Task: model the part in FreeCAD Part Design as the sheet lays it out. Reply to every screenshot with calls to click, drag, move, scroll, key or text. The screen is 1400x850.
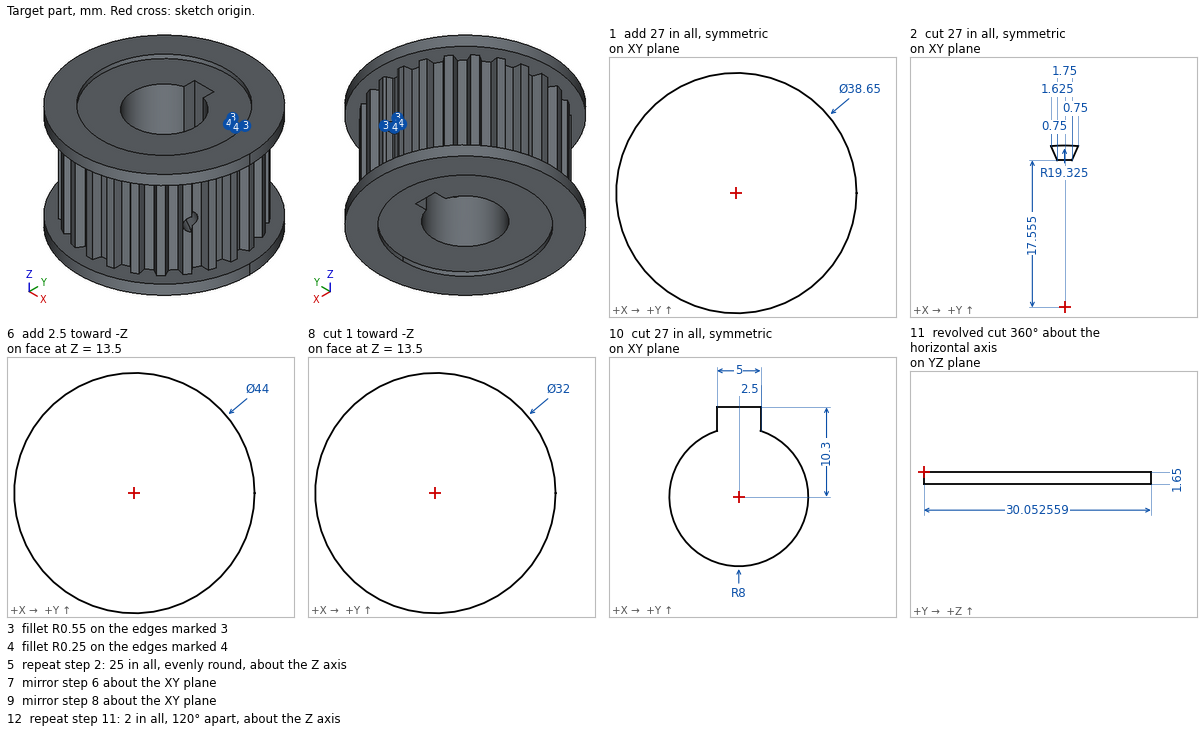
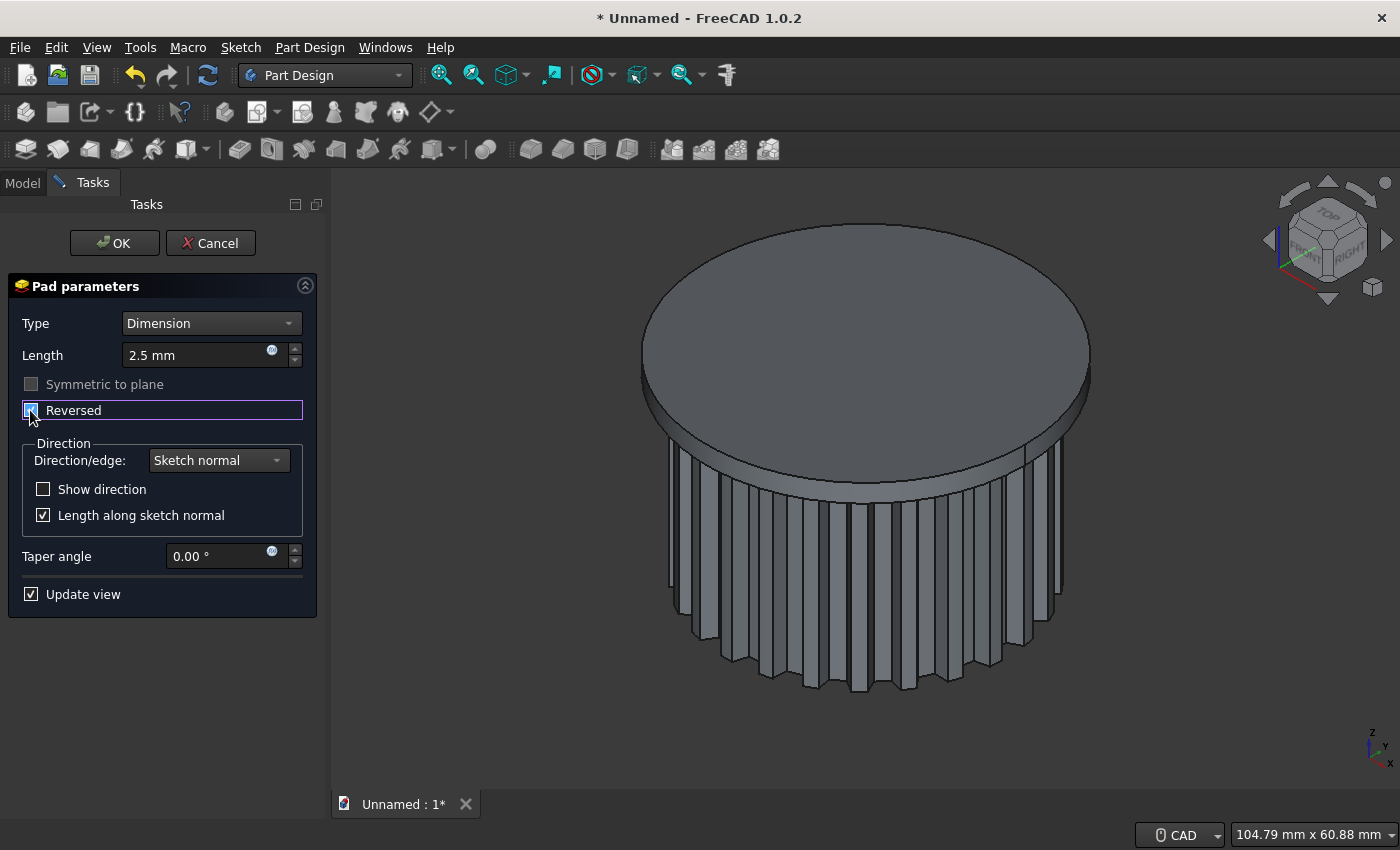
click(115, 243)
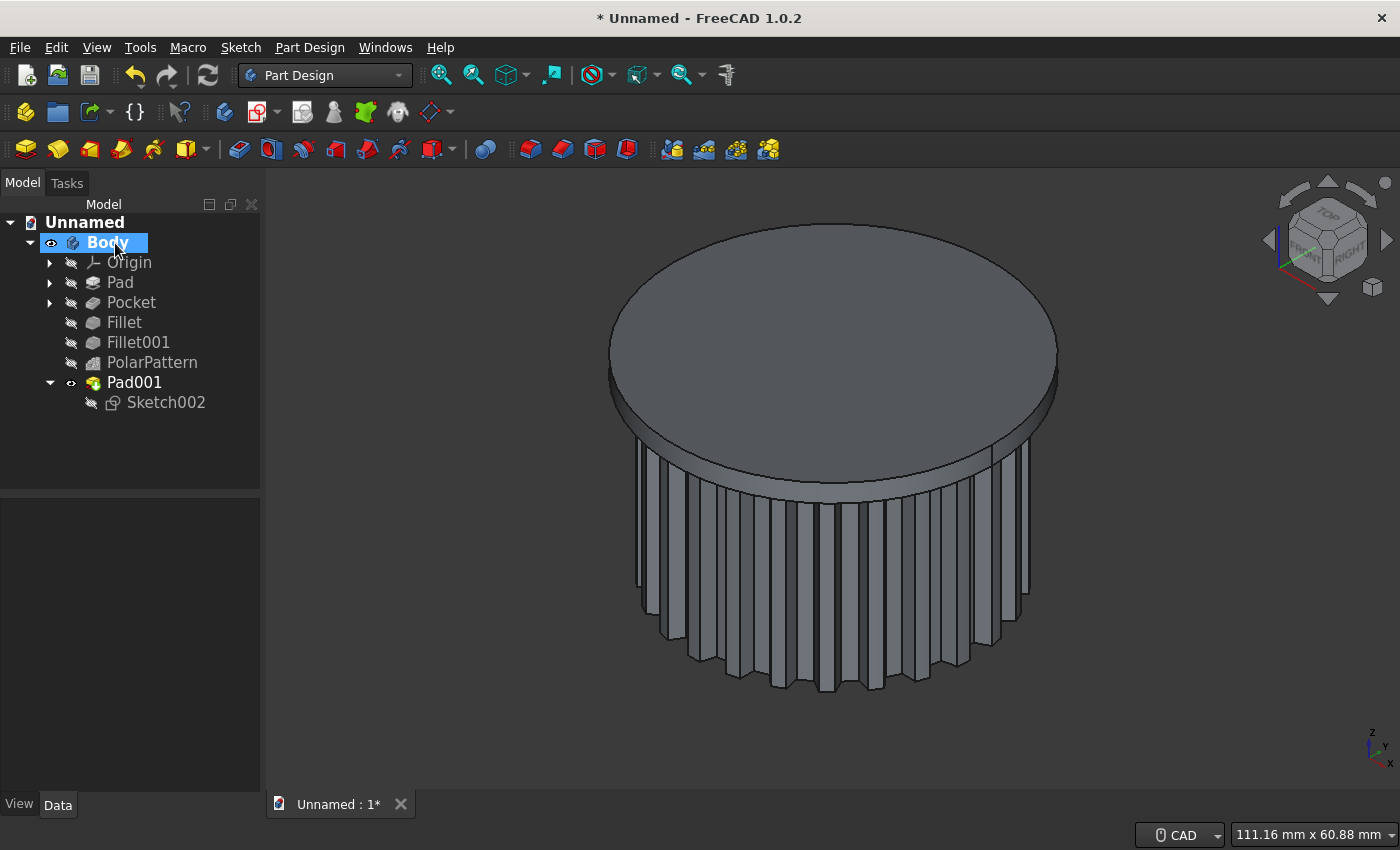
click(116, 383)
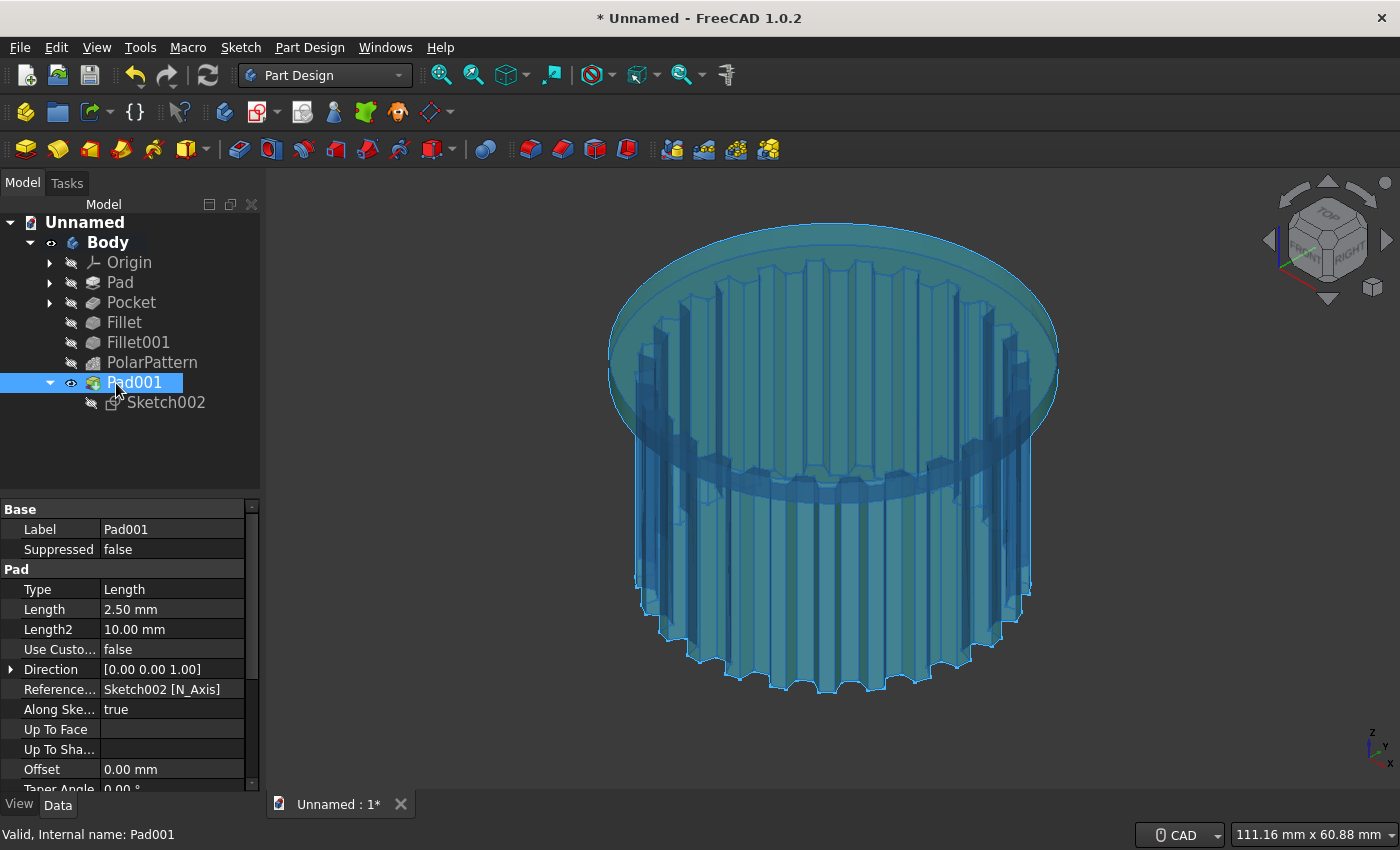
click(672, 150)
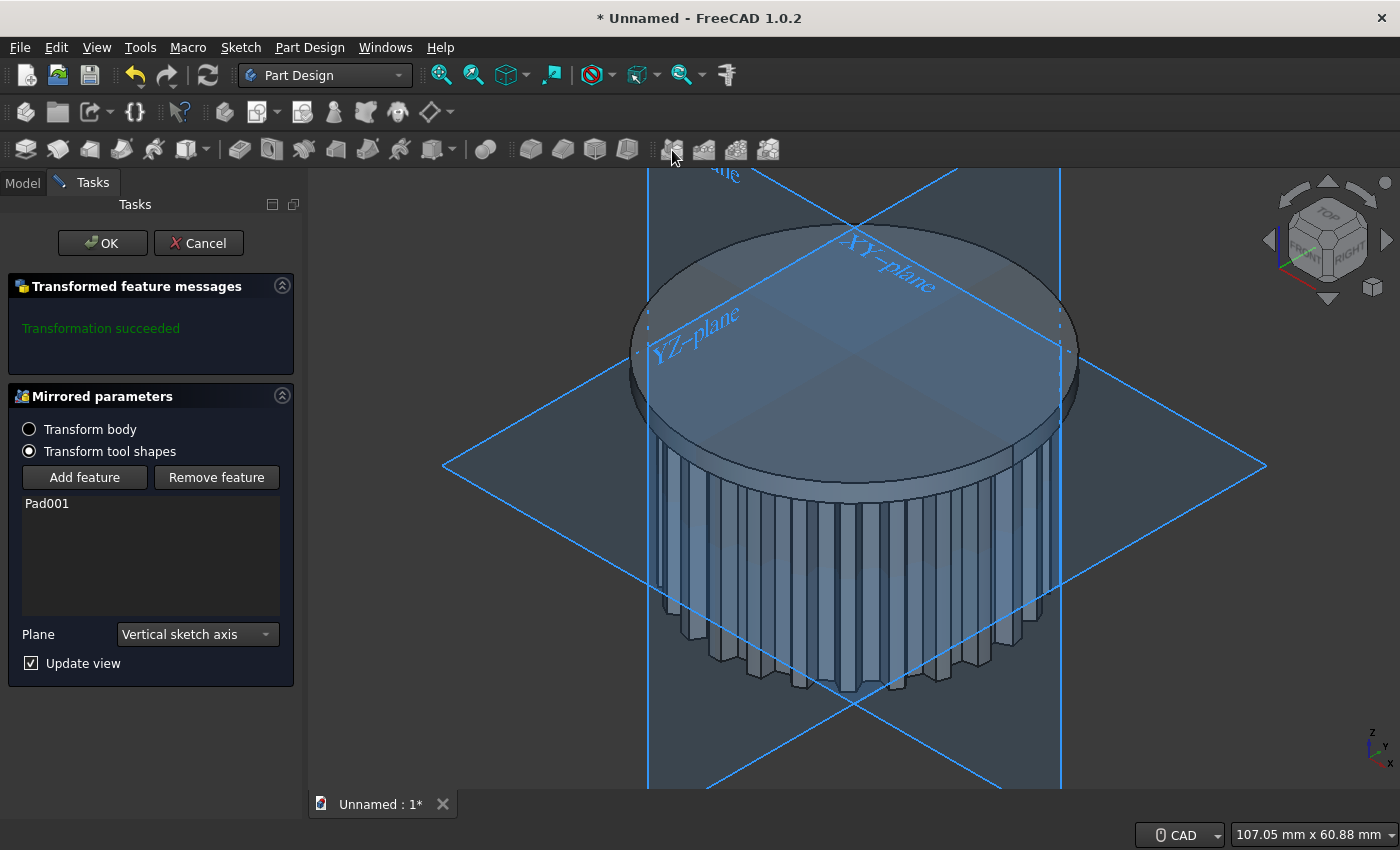
click(198, 634)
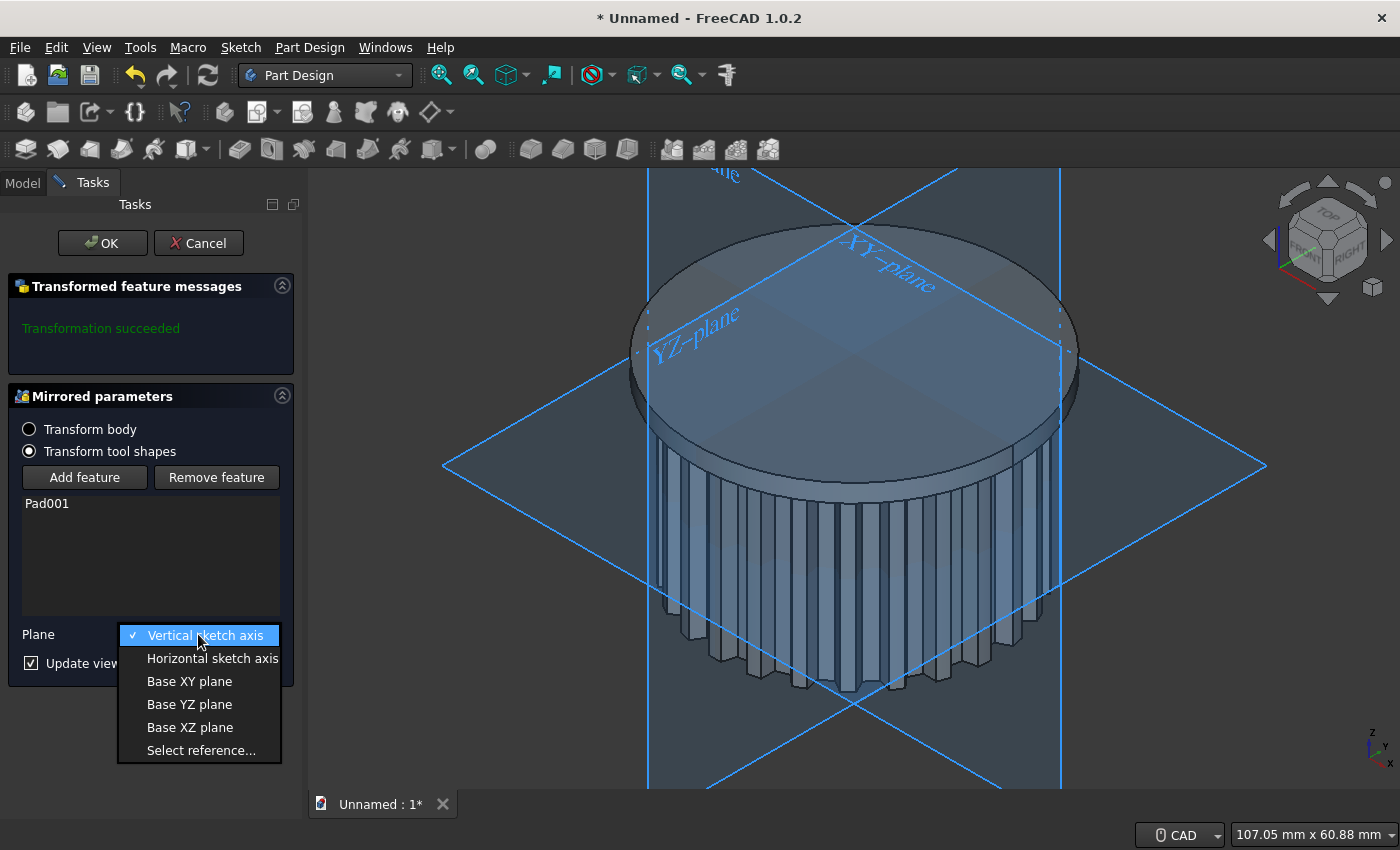
click(198, 682)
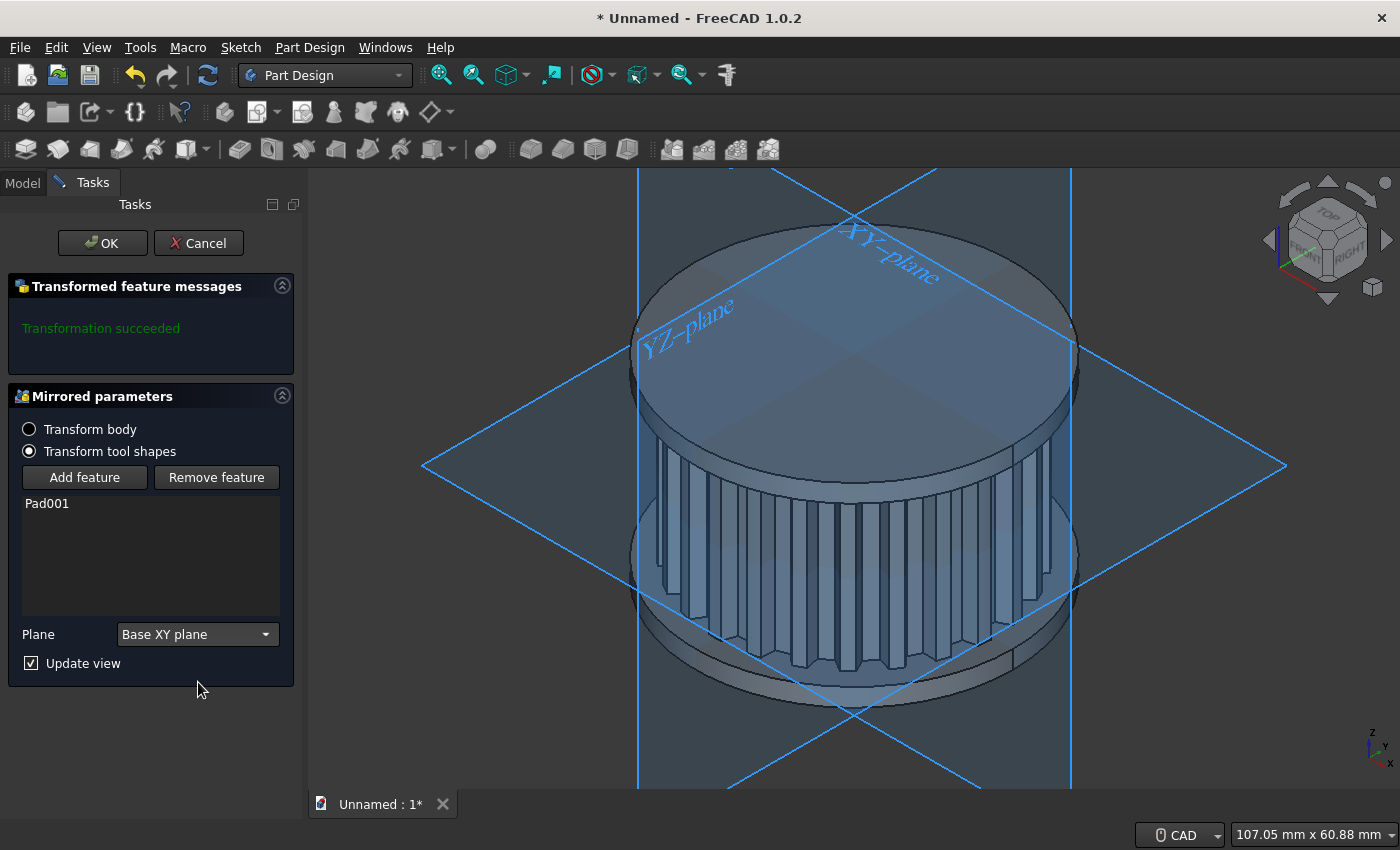
click(103, 243)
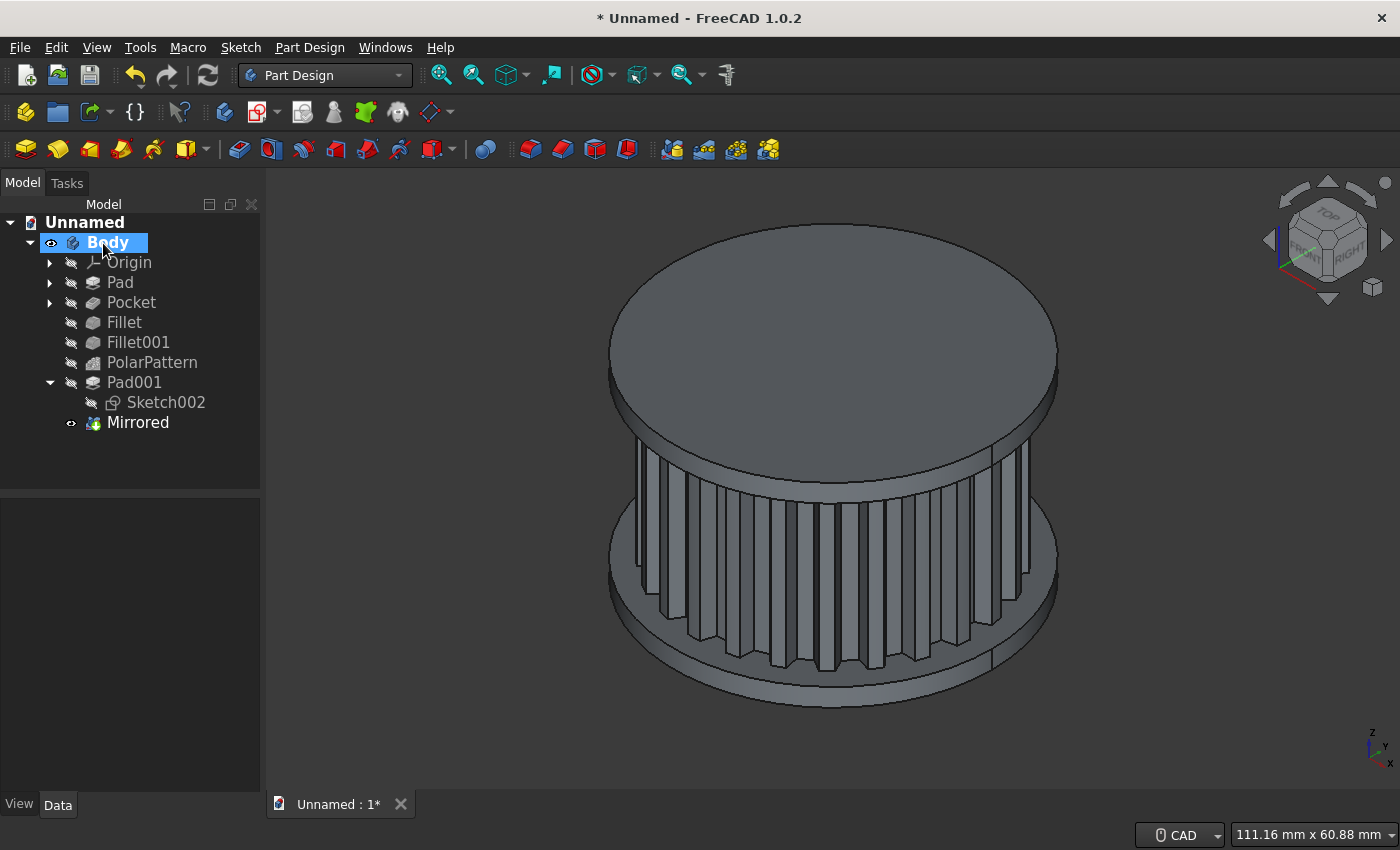
click(833, 352)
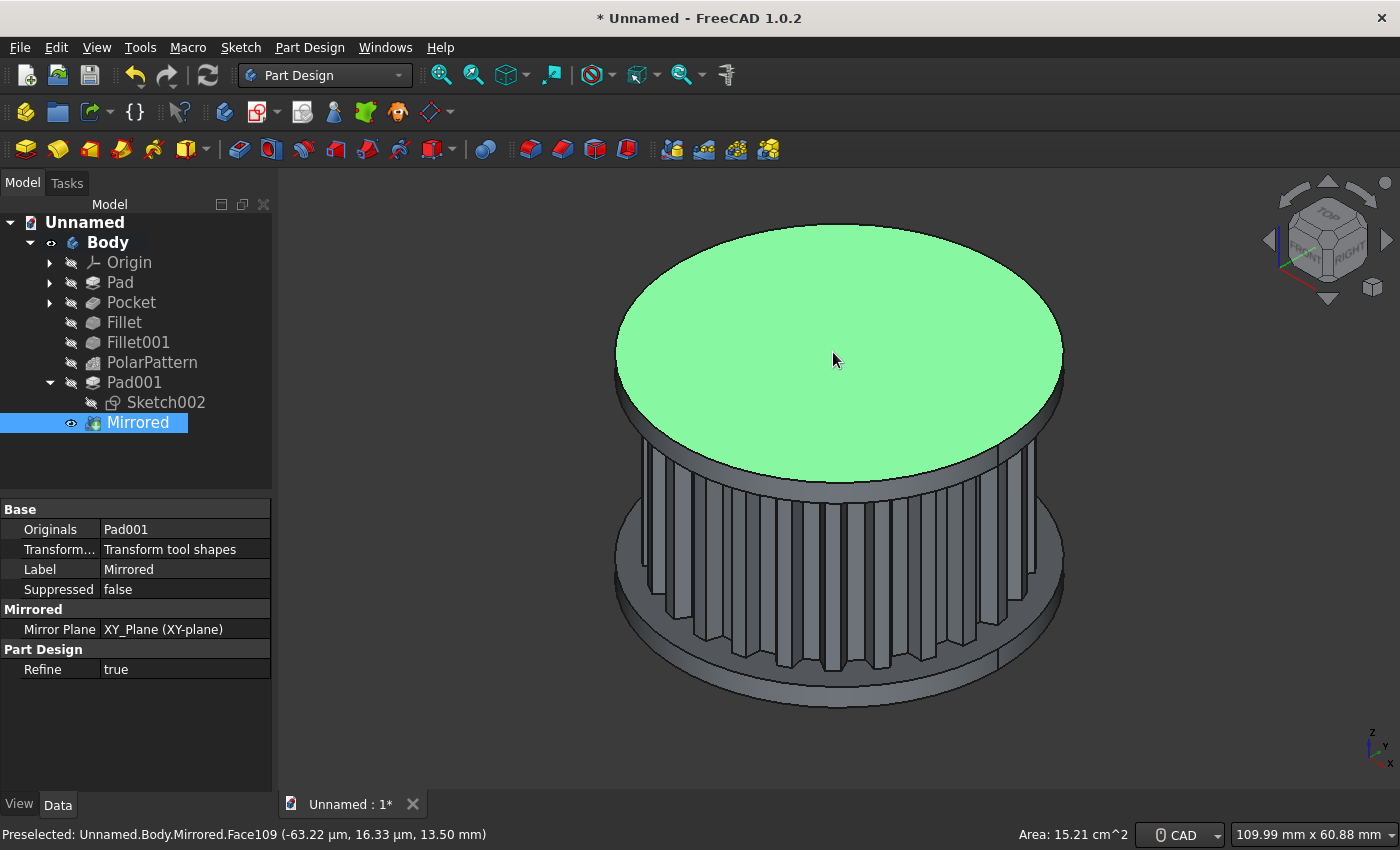
click(258, 112)